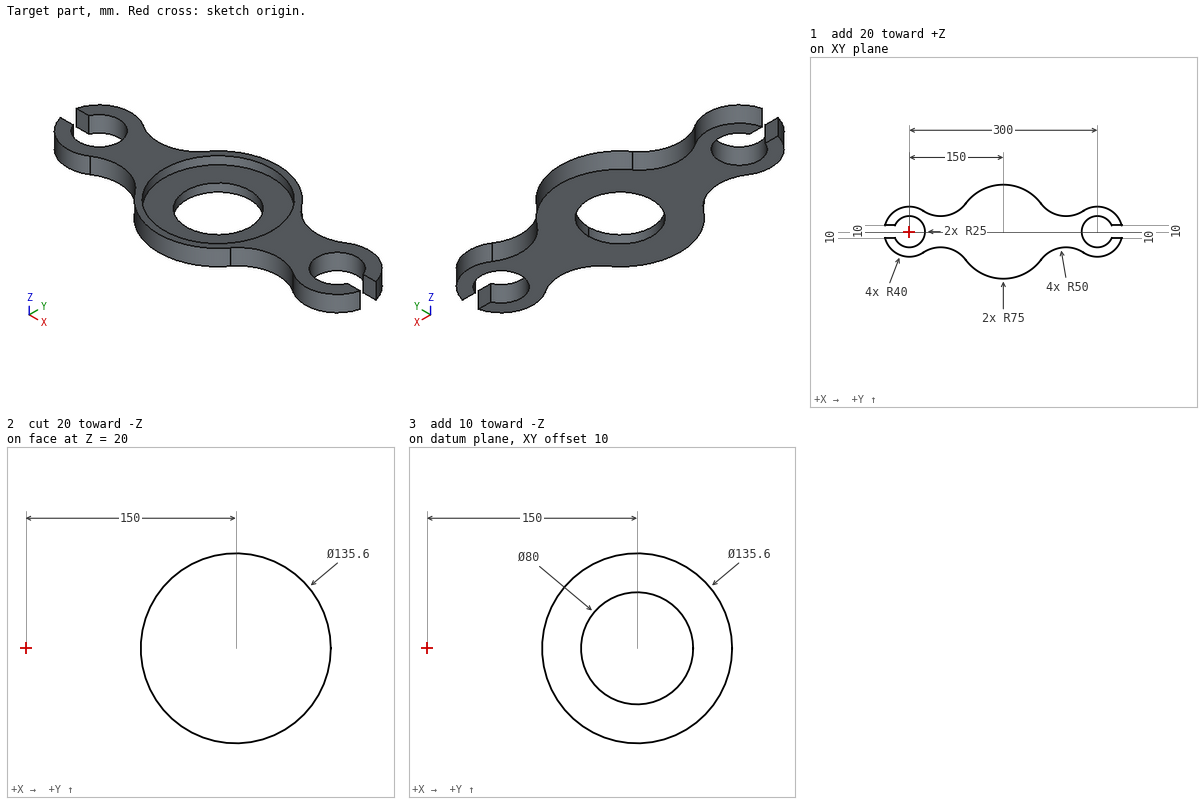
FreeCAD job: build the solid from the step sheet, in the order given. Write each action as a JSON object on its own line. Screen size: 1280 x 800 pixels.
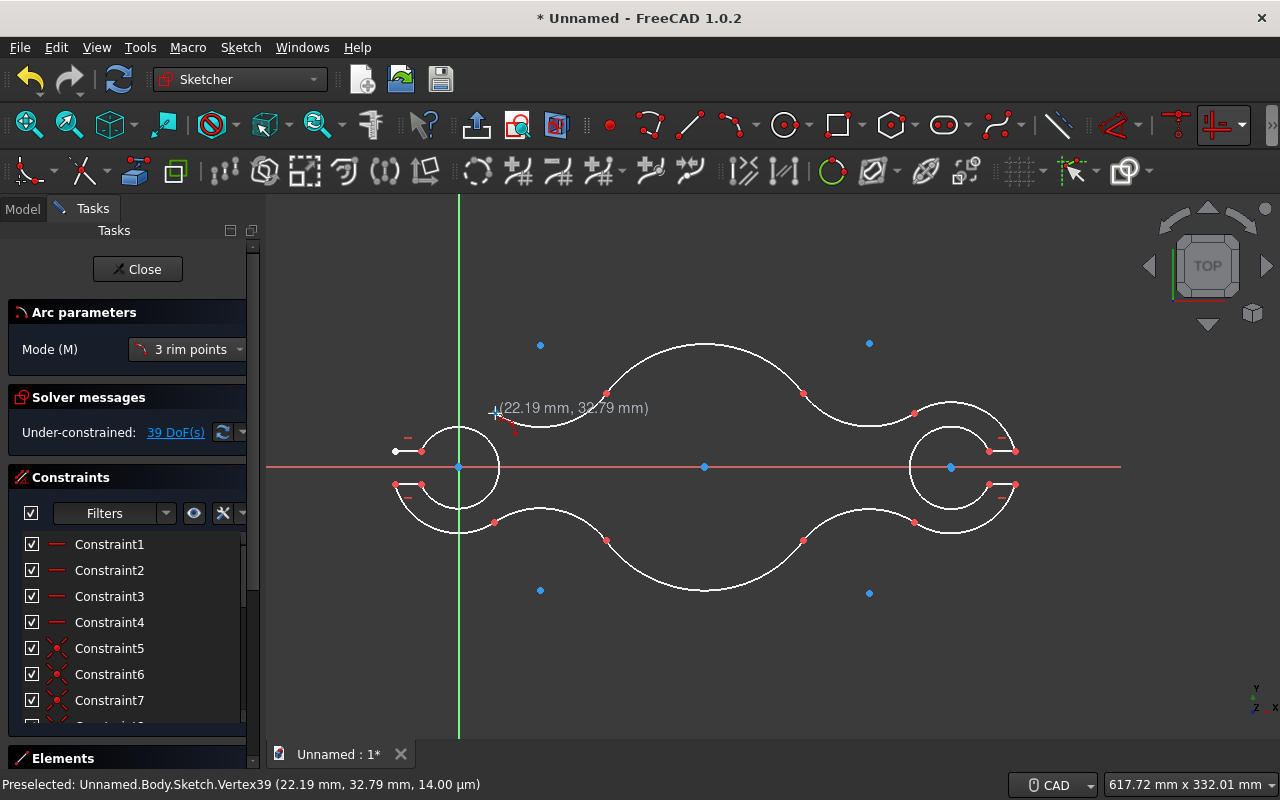
{"action": "scroll", "coordinate": [395, 450], "scroll_direction": "up", "scroll_amount": 2}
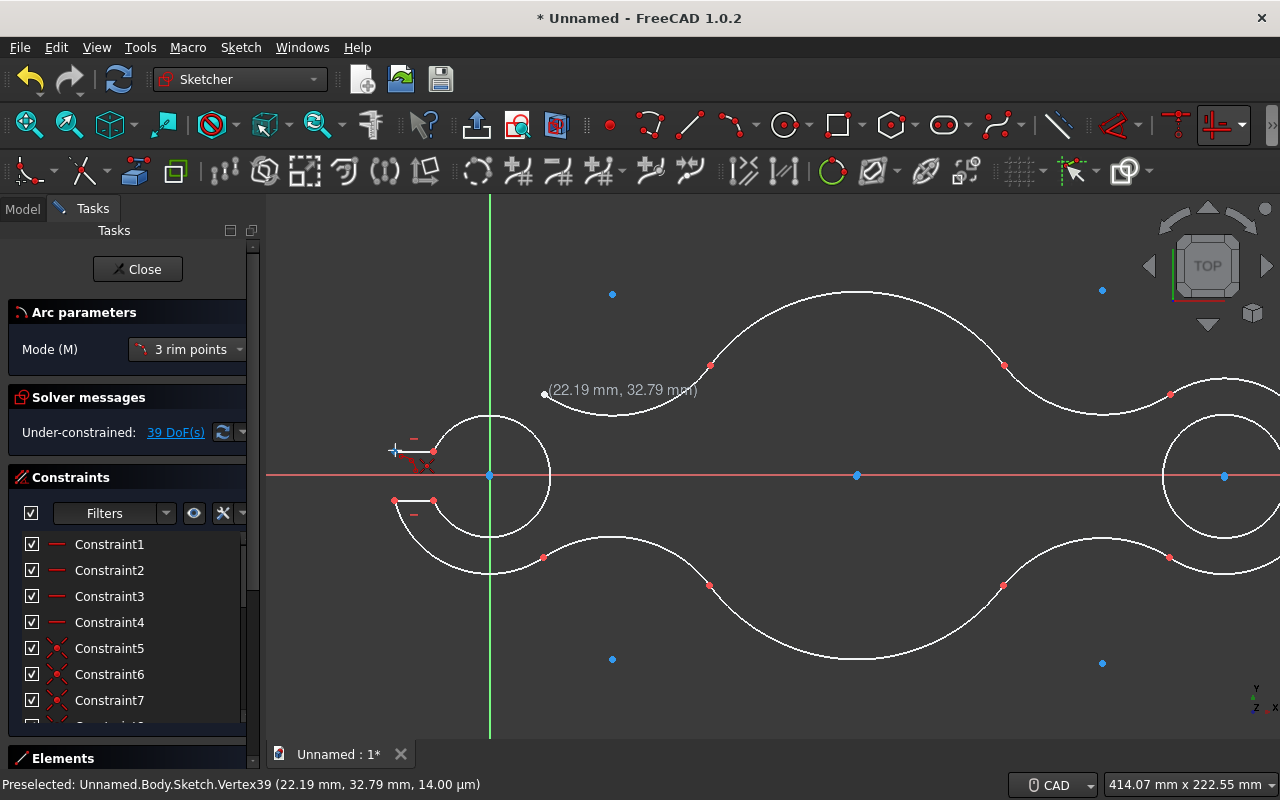
{"action": "left_click", "coordinate": [395, 452]}
{"action": "left_click", "coordinate": [455, 383]}
{"action": "key", "text": "Escape"}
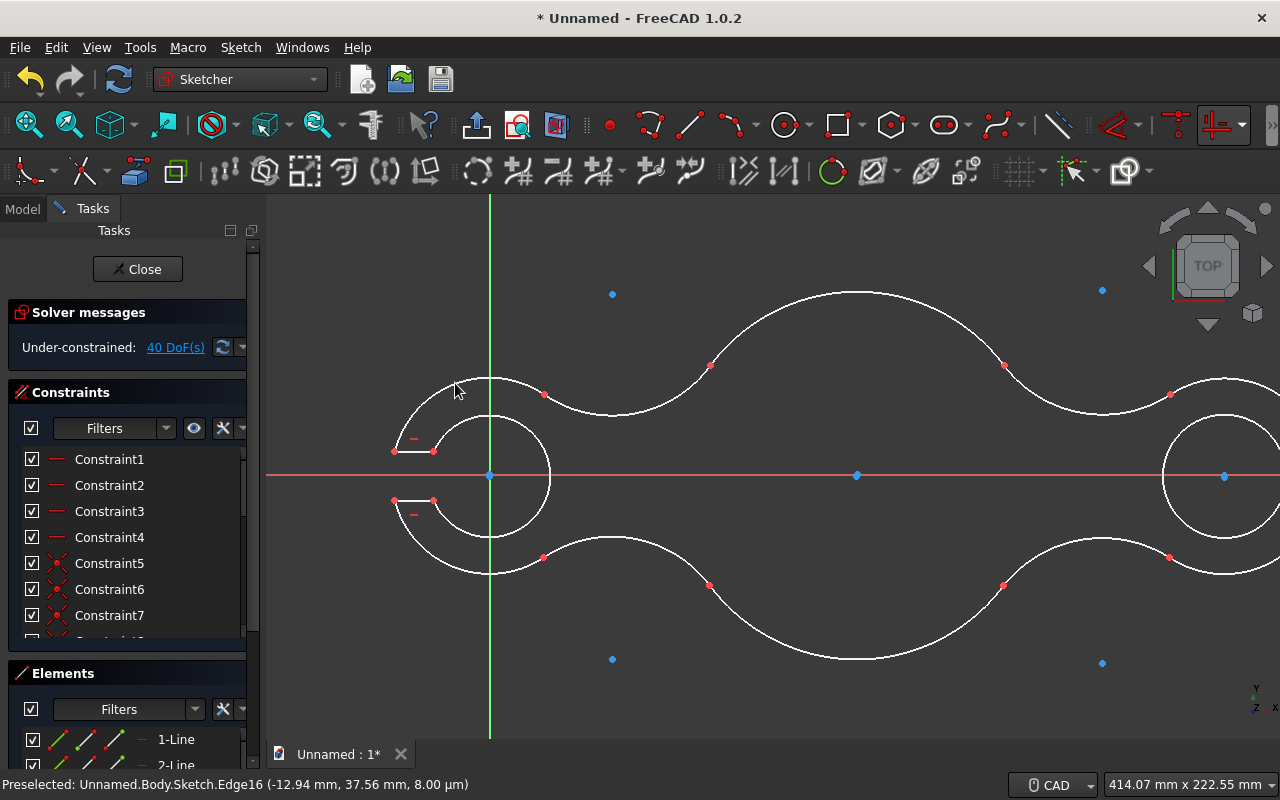
{"action": "left_click", "coordinate": [423, 548]}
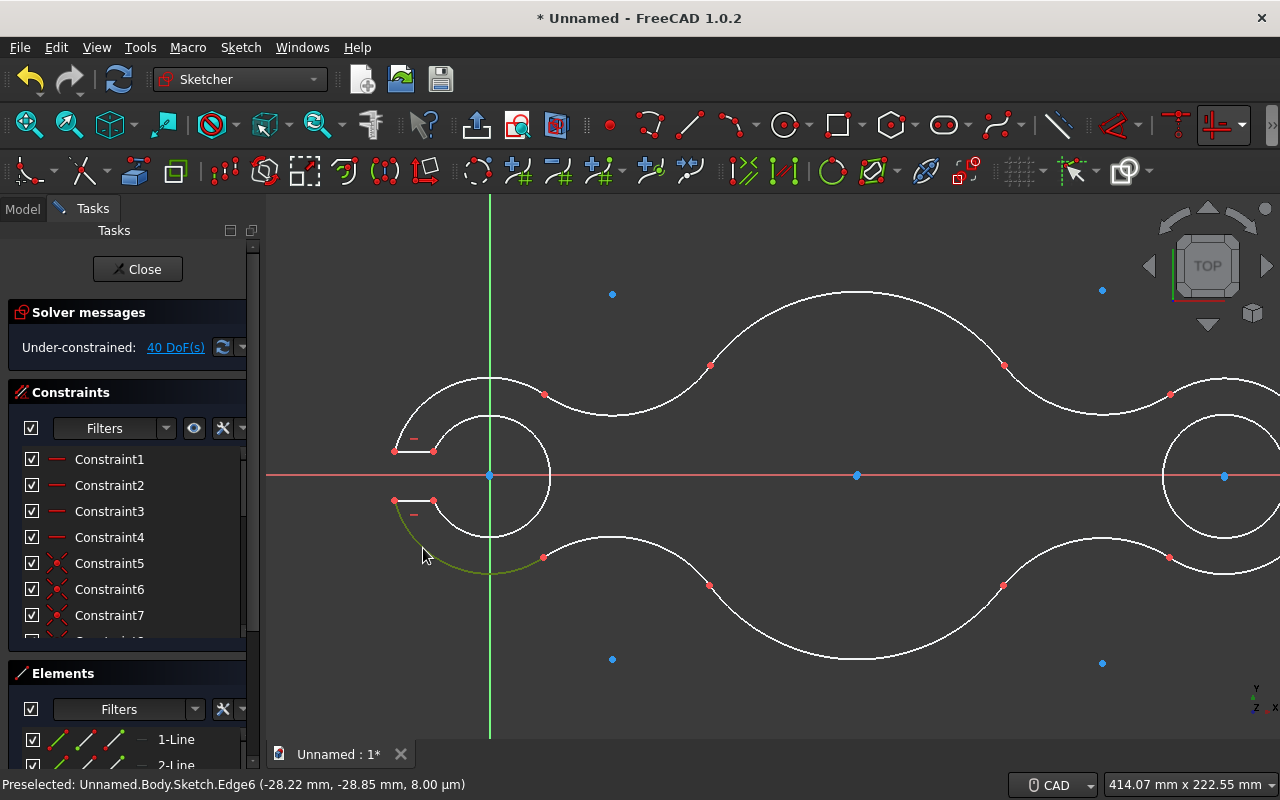
{"action": "left_click", "coordinate": [667, 550]}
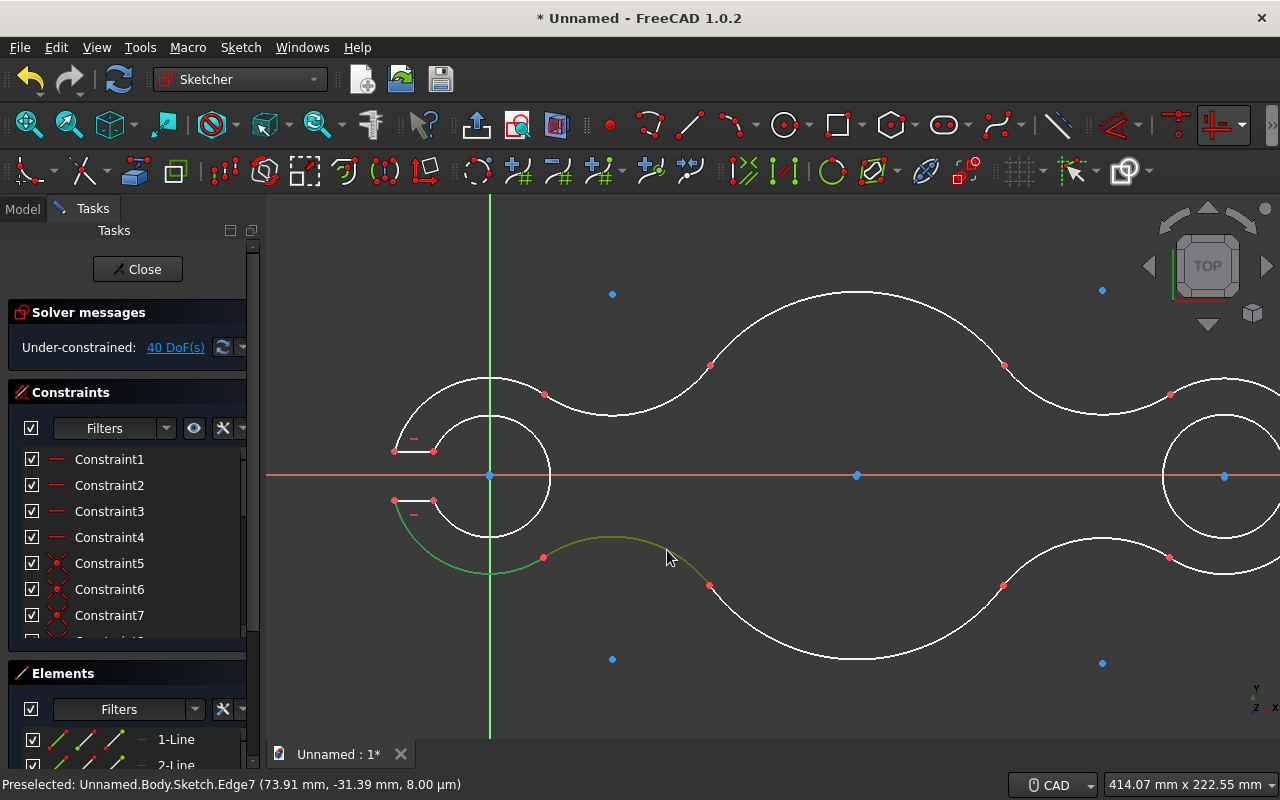
{"action": "key", "text": "t"}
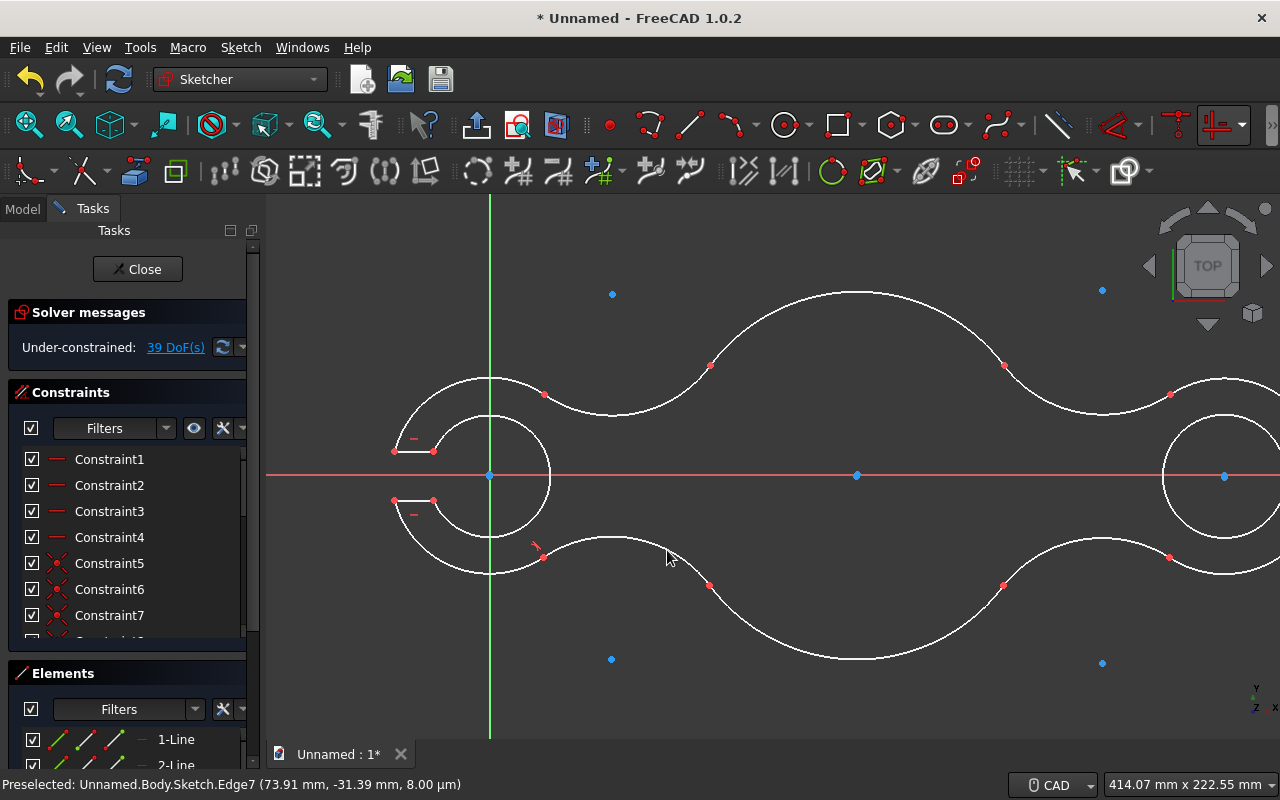
{"action": "left_click", "coordinate": [668, 550]}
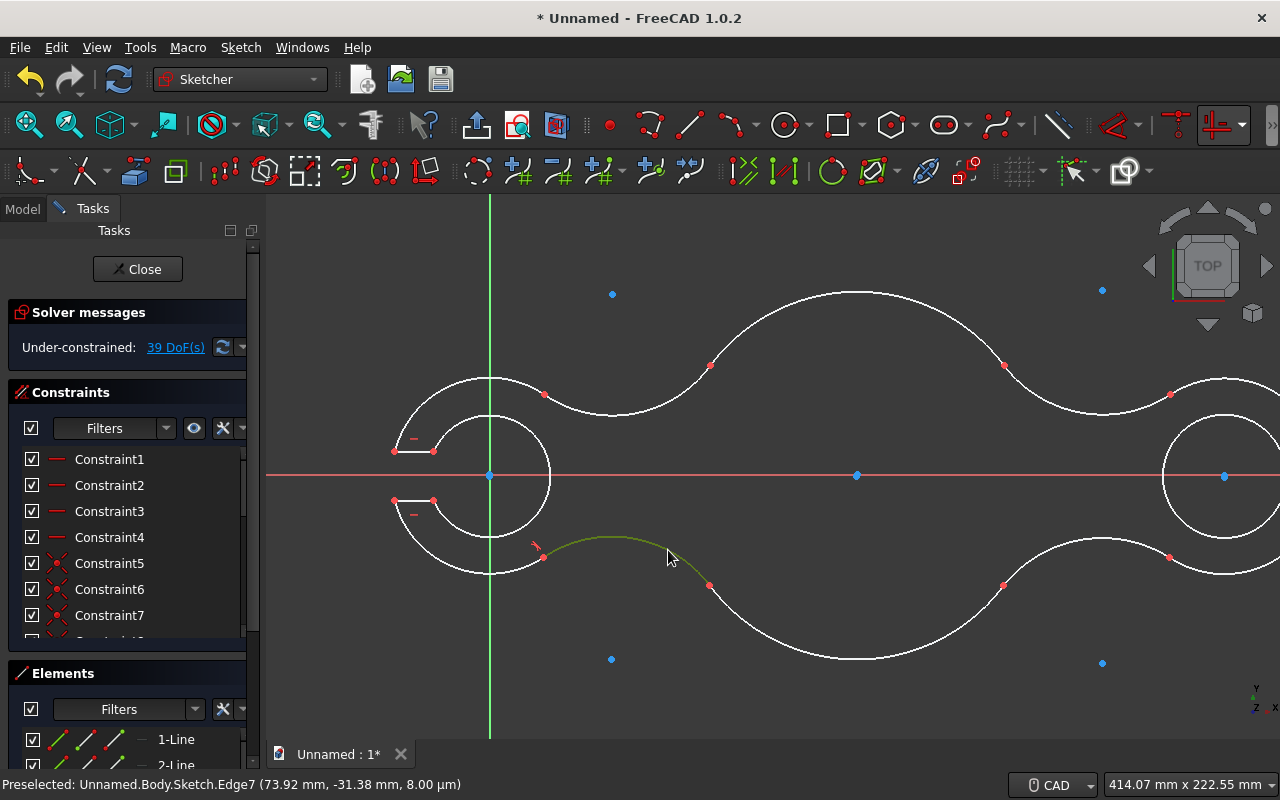
{"action": "left_click", "coordinate": [790, 647]}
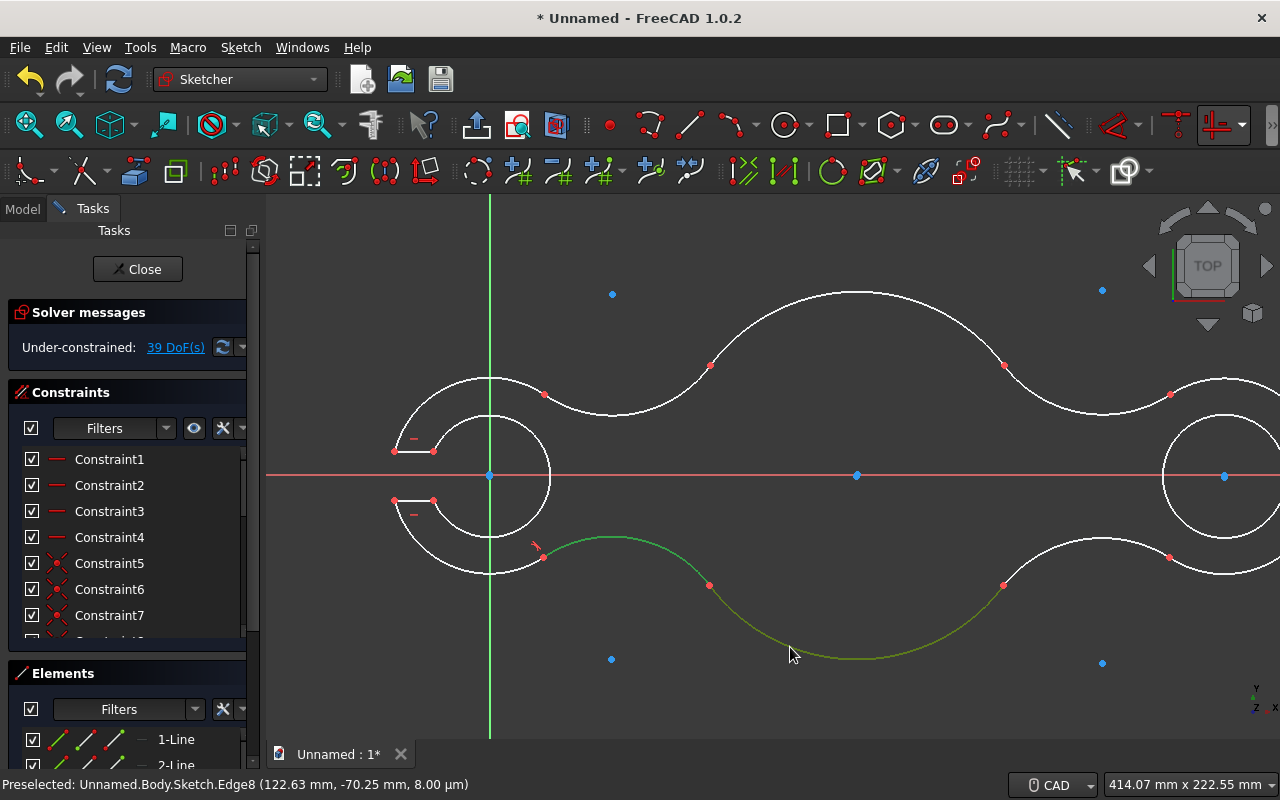
{"action": "key", "text": "t"}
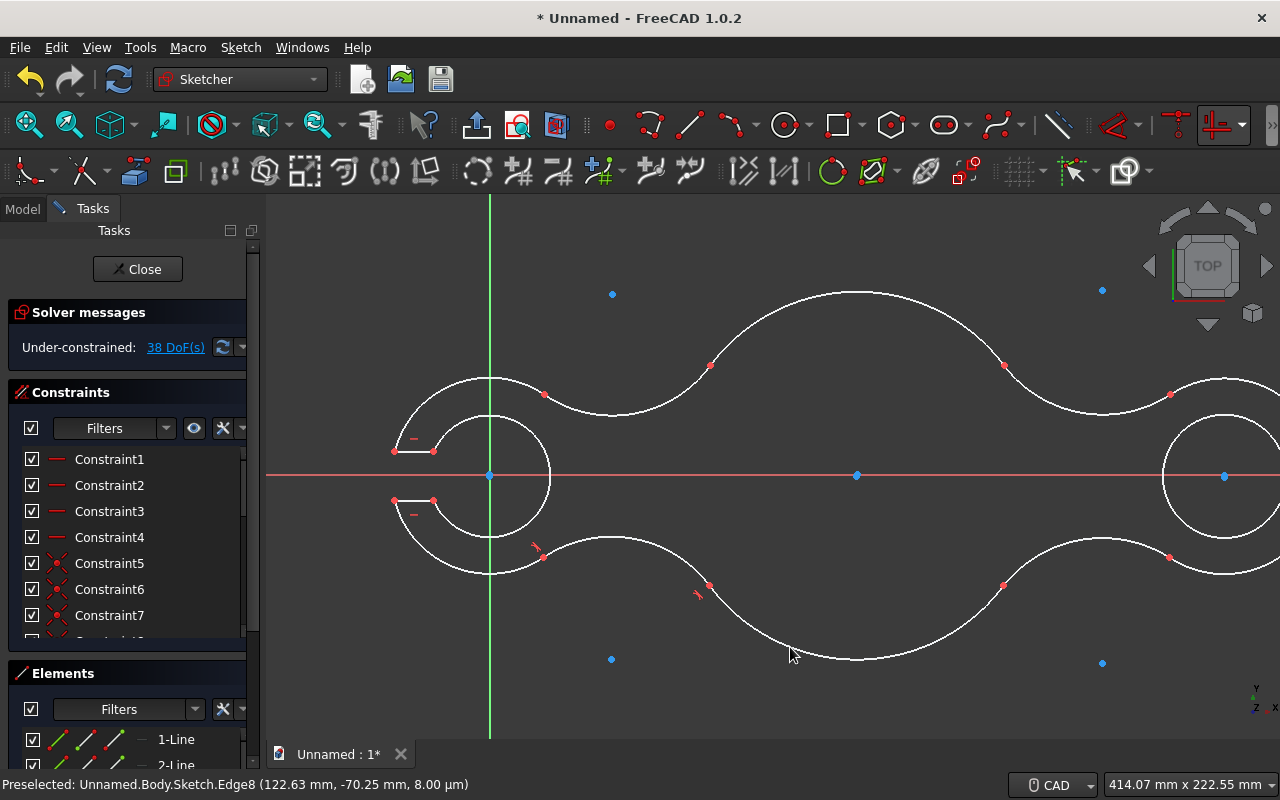
{"action": "left_click", "coordinate": [790, 647]}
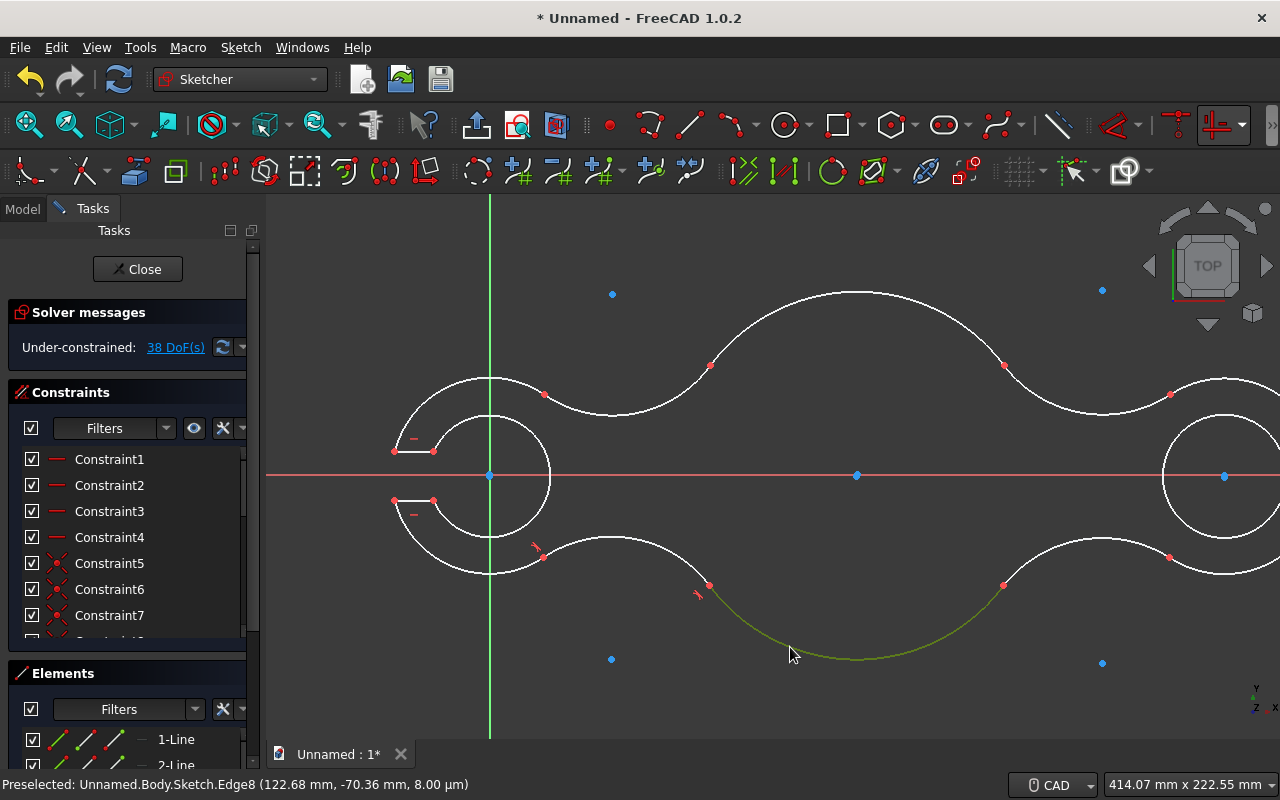
{"action": "left_click", "coordinate": [1046, 551]}